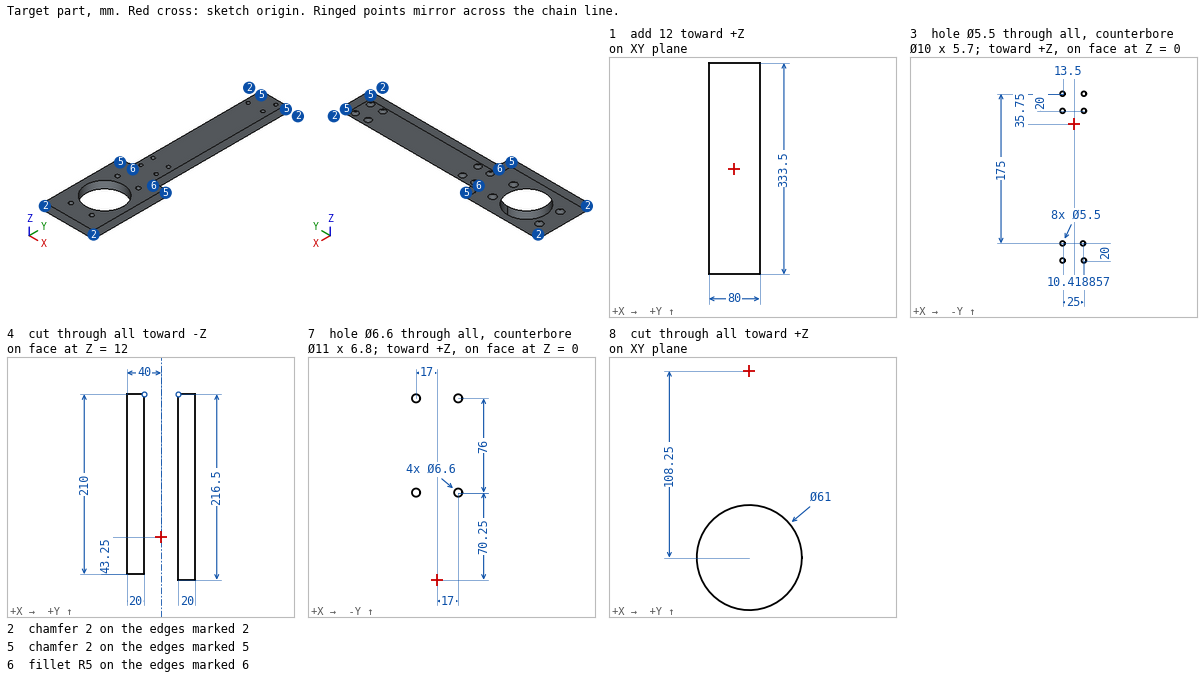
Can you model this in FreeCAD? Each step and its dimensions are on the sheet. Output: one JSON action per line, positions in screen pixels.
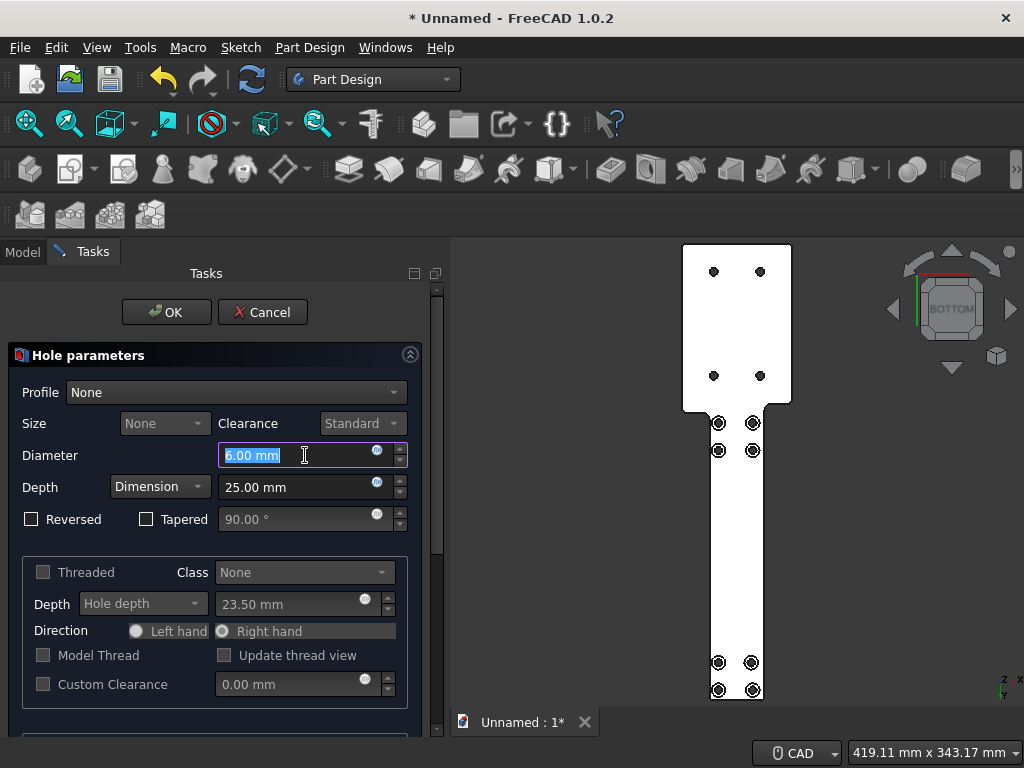
{"action": "type", "text": "6.6"}
{"action": "key", "text": "Tab"}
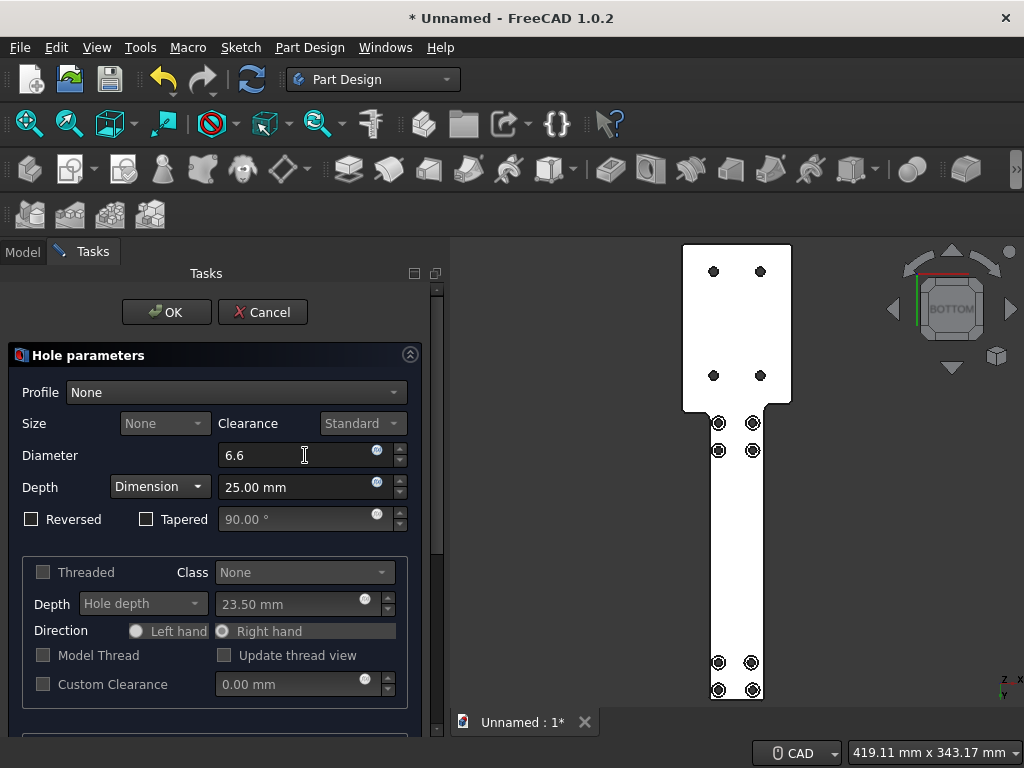
{"action": "left_click", "coordinate": [161, 486]}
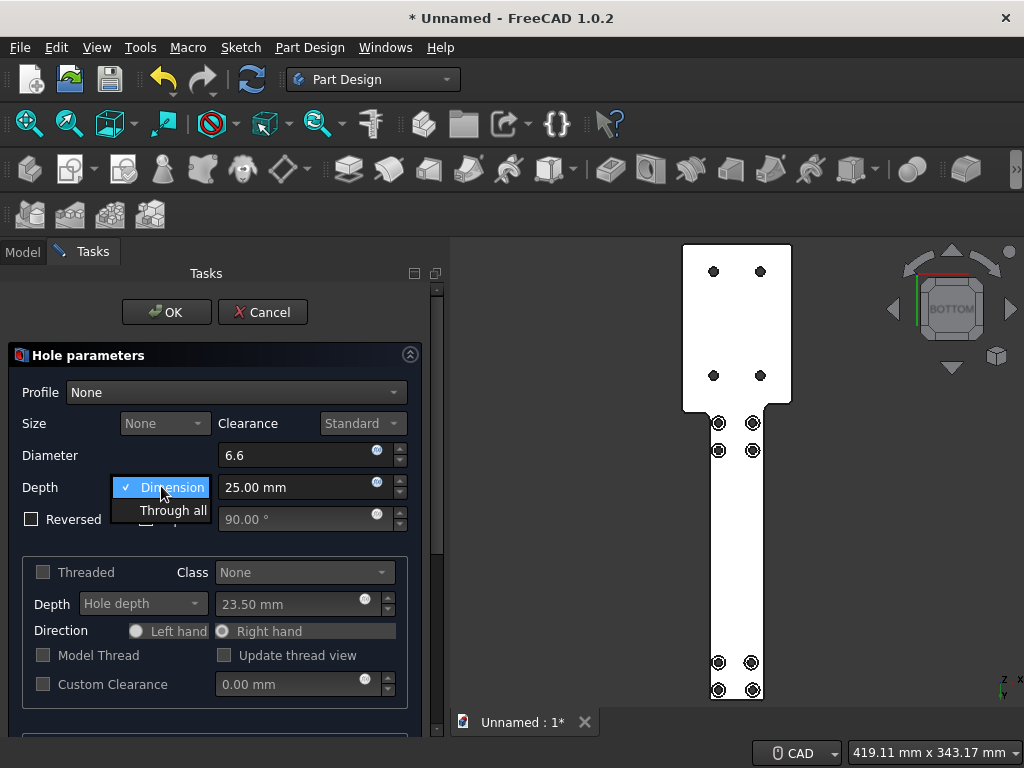
{"action": "left_click", "coordinate": [160, 510]}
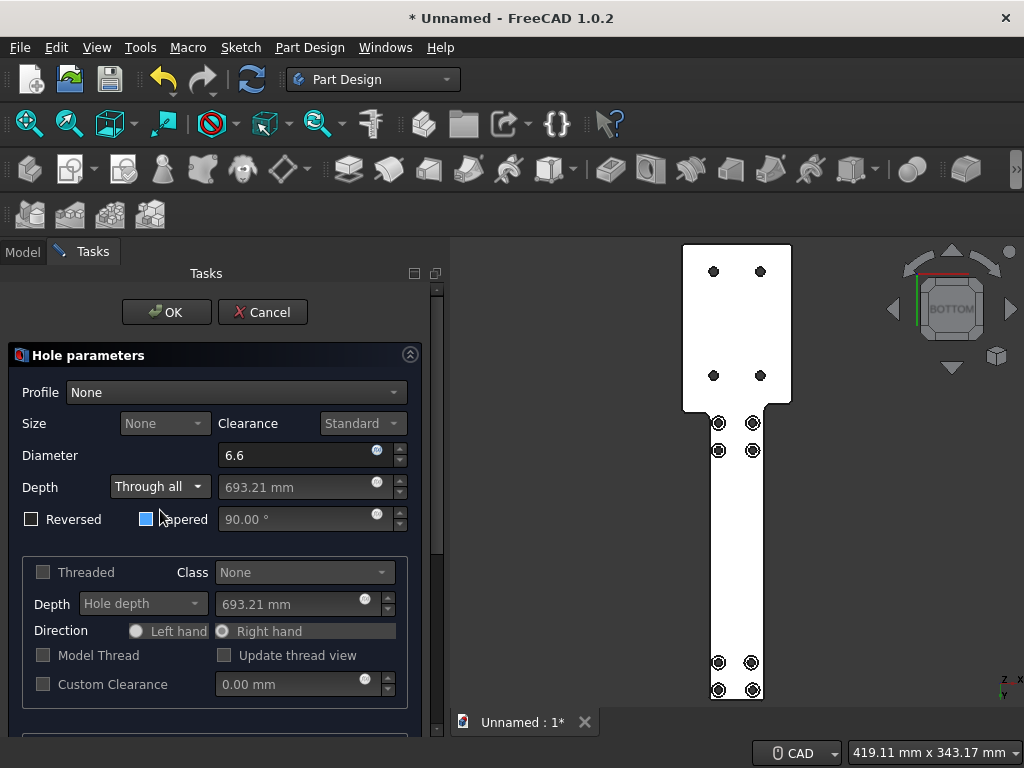
{"action": "scroll", "coordinate": [437, 510], "scroll_direction": "down", "scroll_amount": 2}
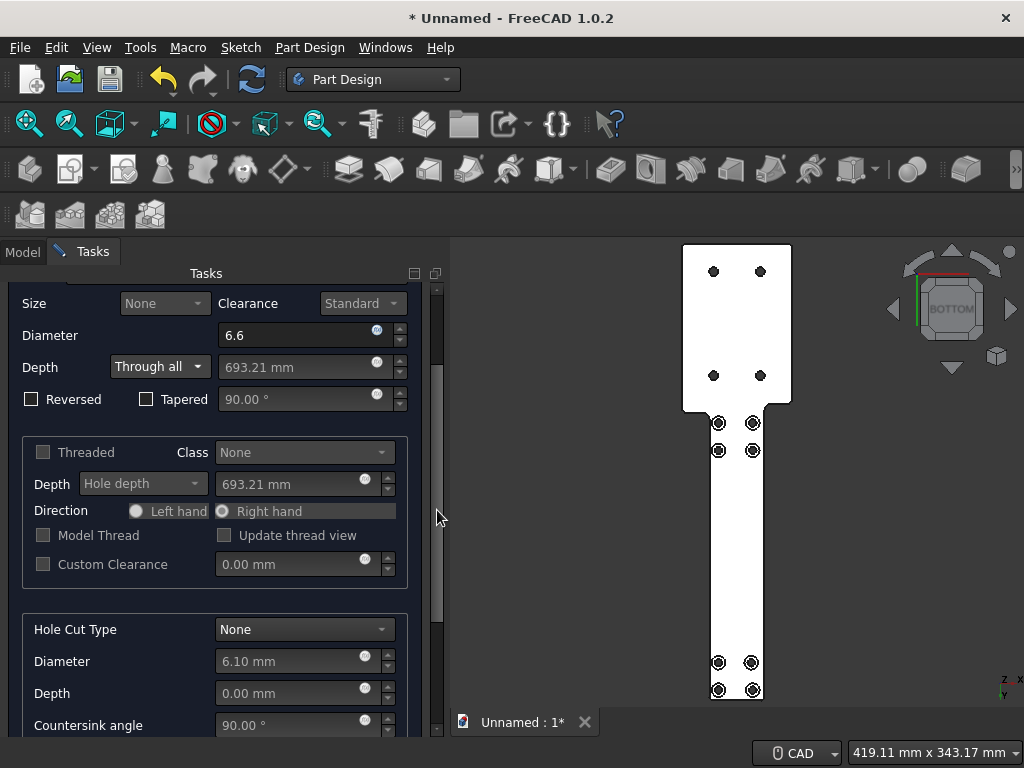
{"action": "left_click", "coordinate": [306, 630]}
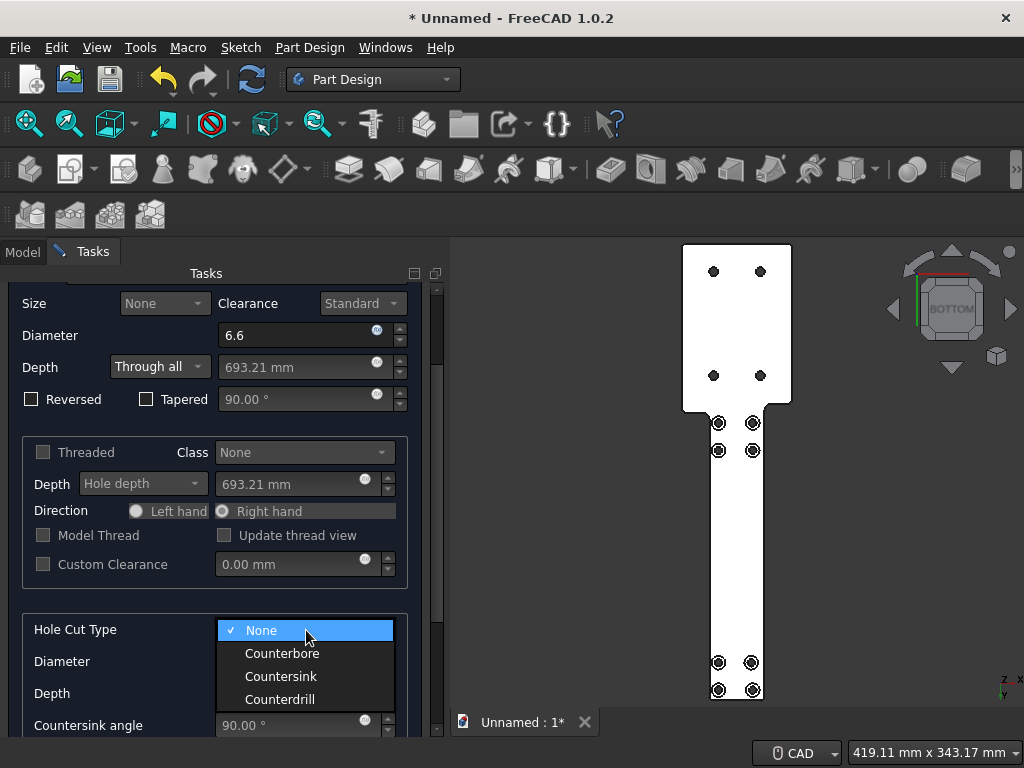
{"action": "left_click", "coordinate": [304, 654]}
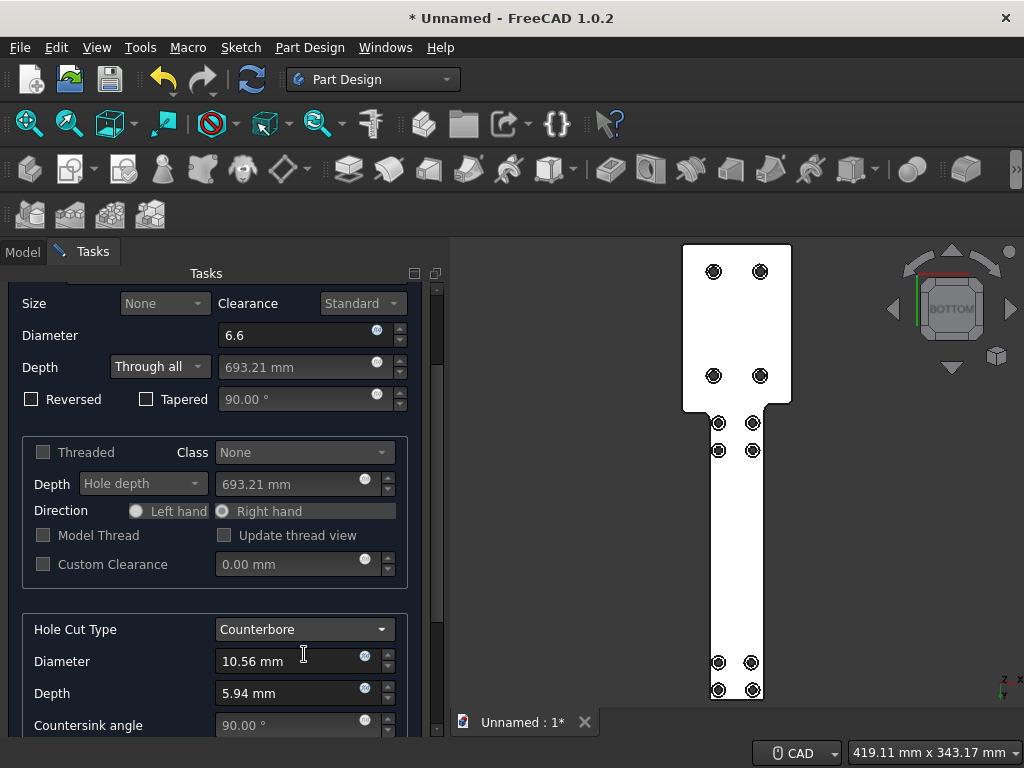
{"action": "triple_click", "coordinate": [298, 661]}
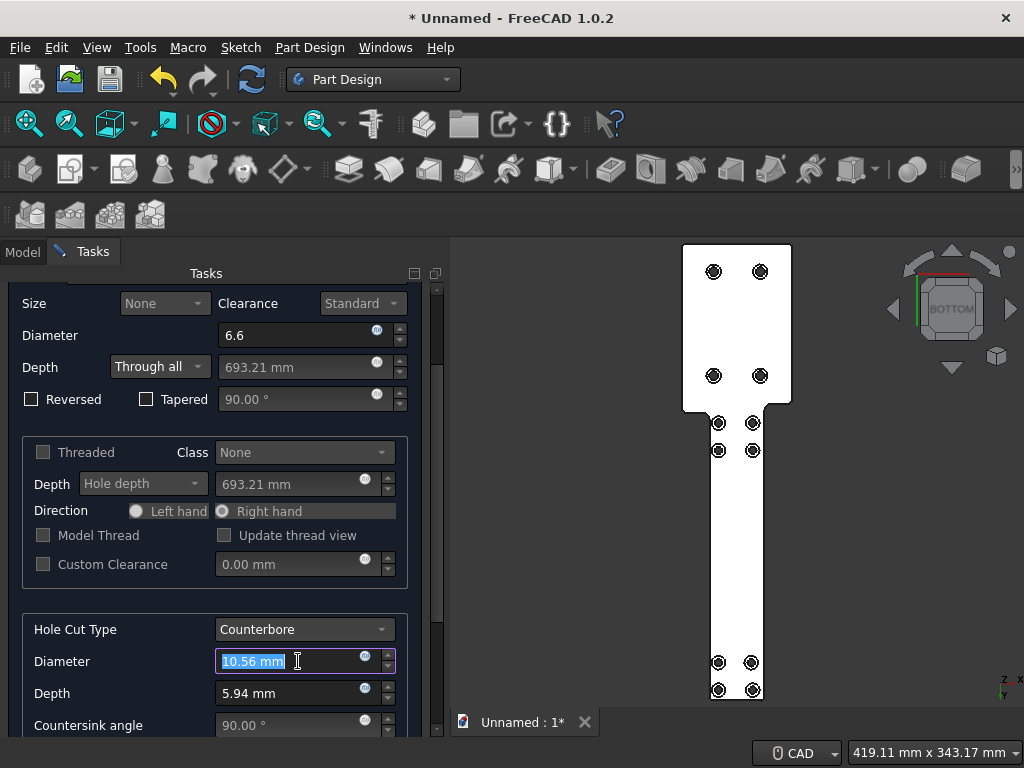
{"action": "type", "text": "11"}
{"action": "key", "text": "Tab"}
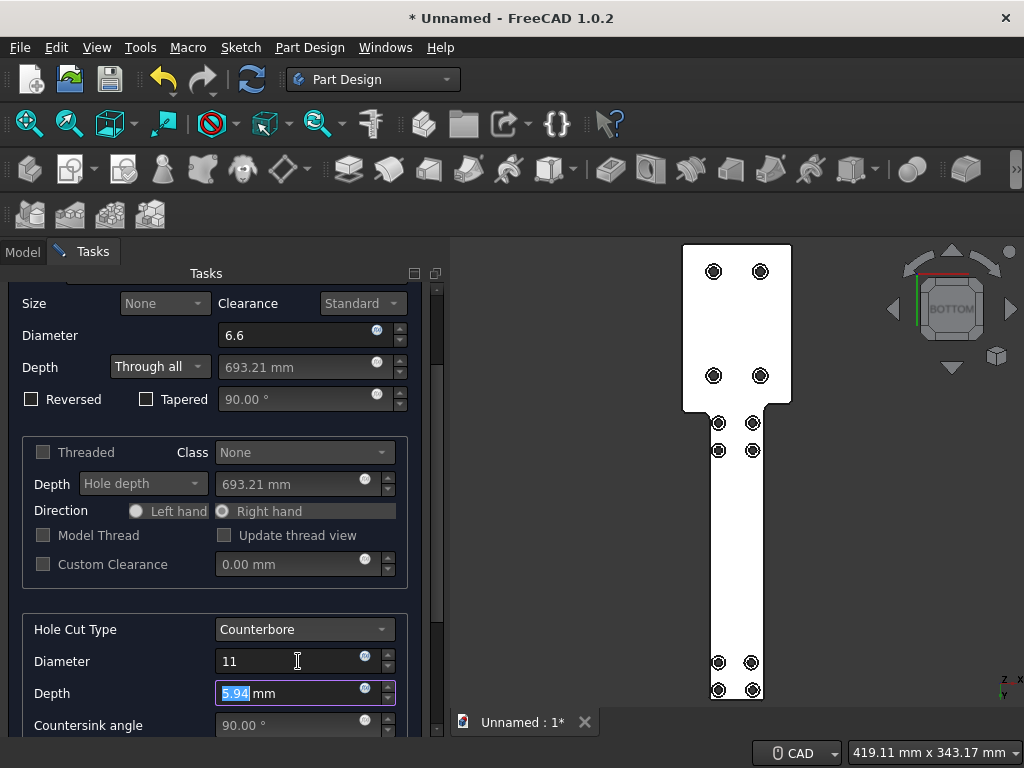
{"action": "type", "text": "6.8"}
{"action": "key", "text": "Tab"}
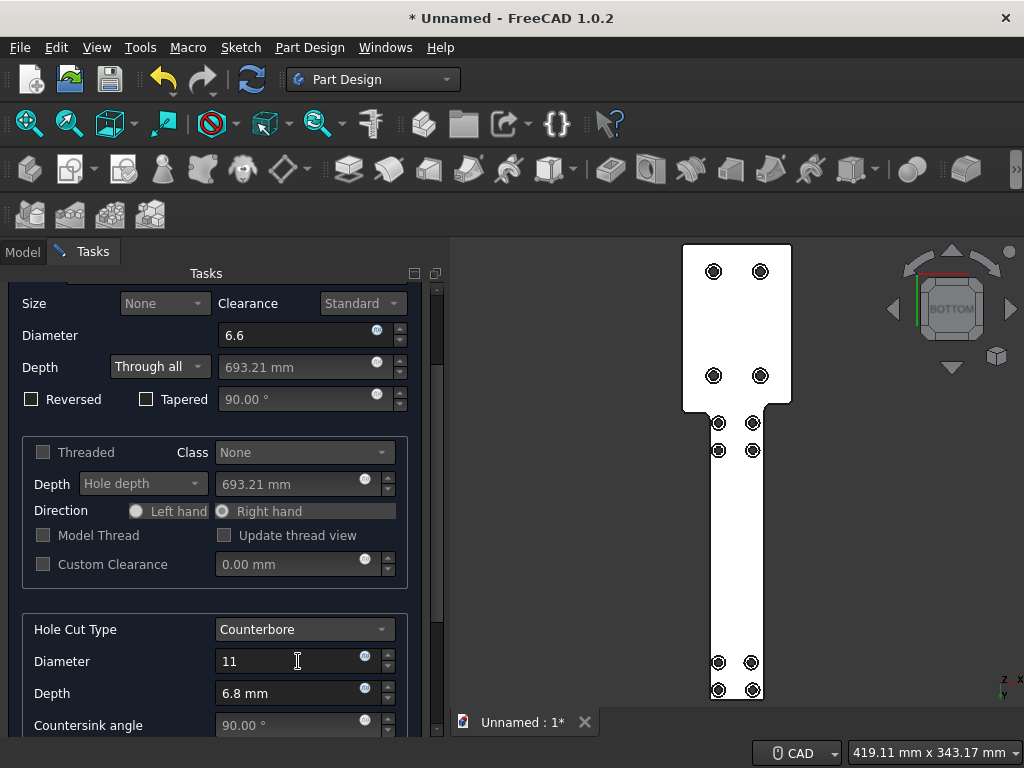
{"action": "scroll", "coordinate": [437, 510], "scroll_direction": "up", "scroll_amount": 3}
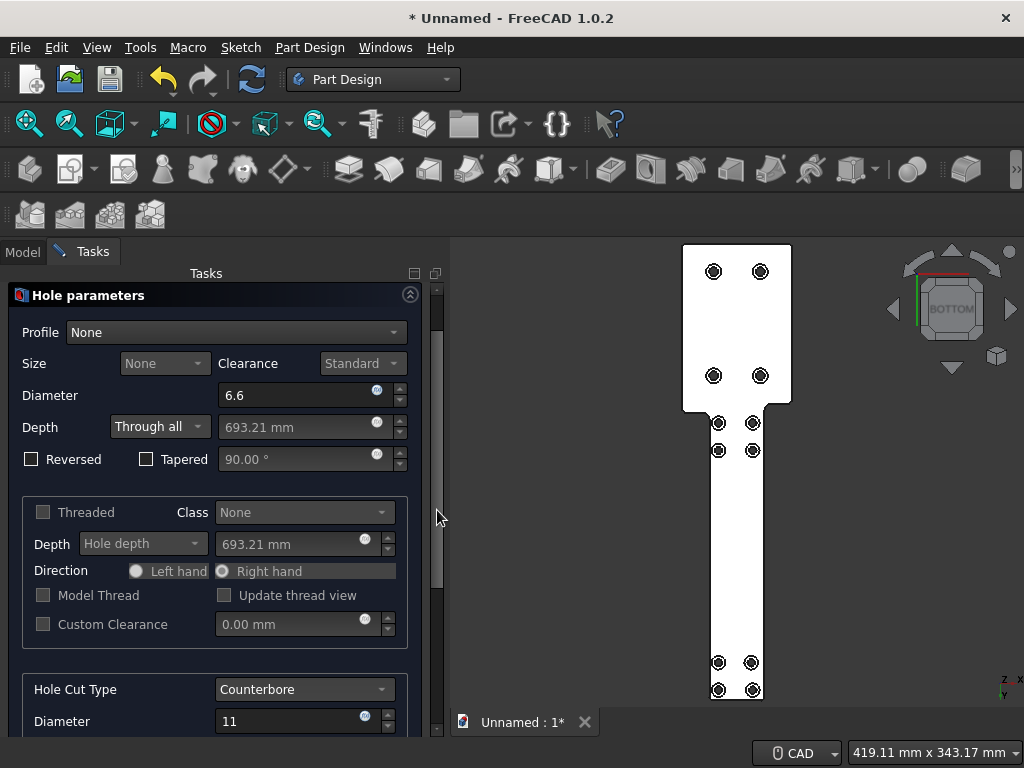
{"action": "left_click", "coordinate": [167, 312]}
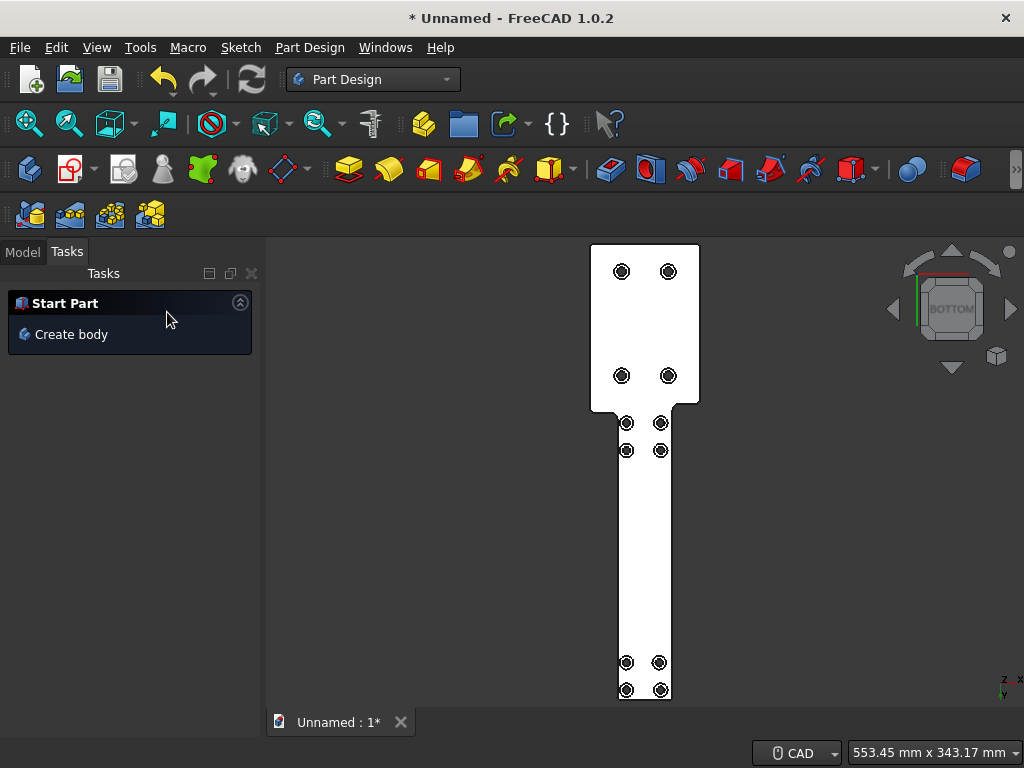
{"action": "left_click", "coordinate": [70, 170]}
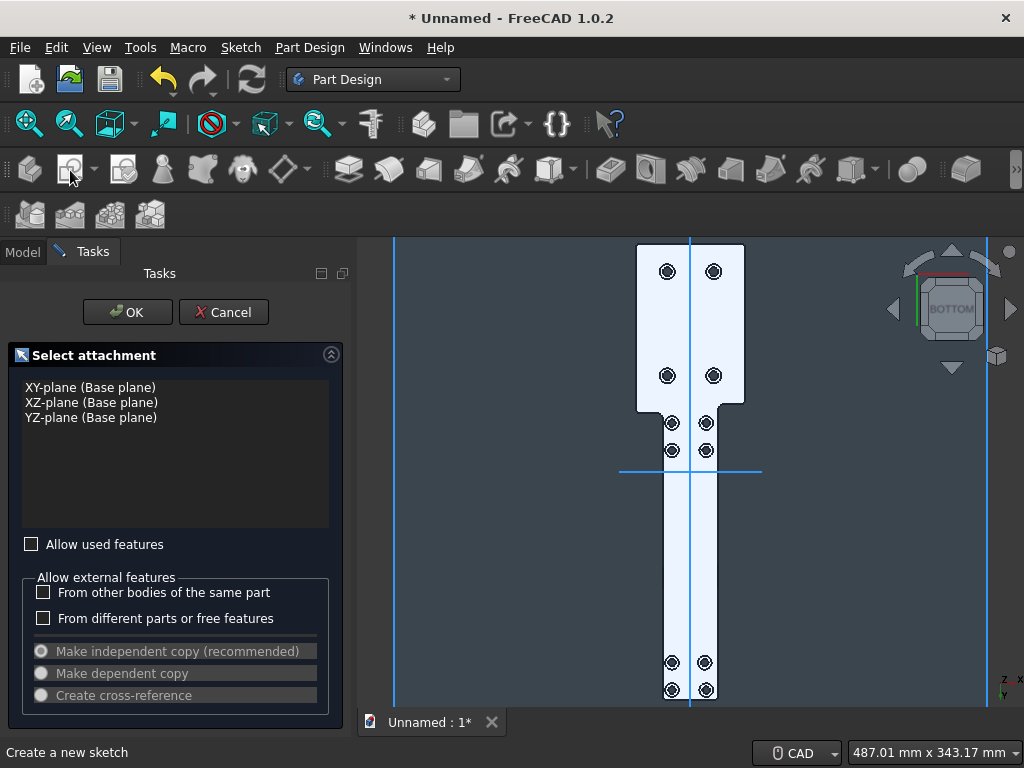
{"action": "left_click", "coordinate": [82, 388]}